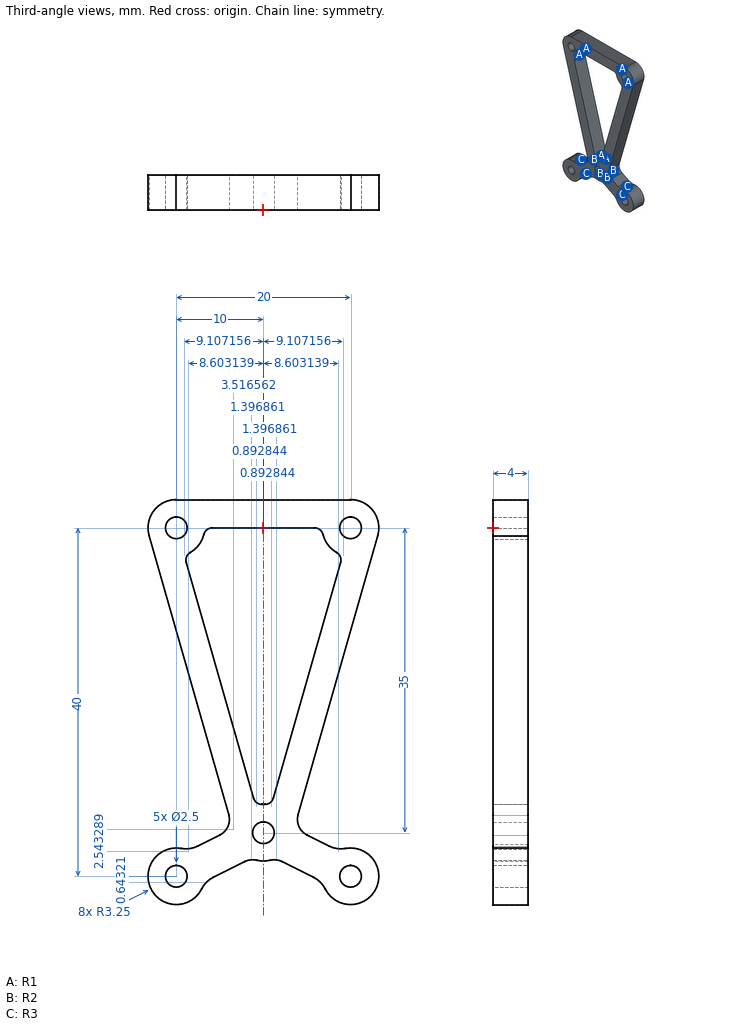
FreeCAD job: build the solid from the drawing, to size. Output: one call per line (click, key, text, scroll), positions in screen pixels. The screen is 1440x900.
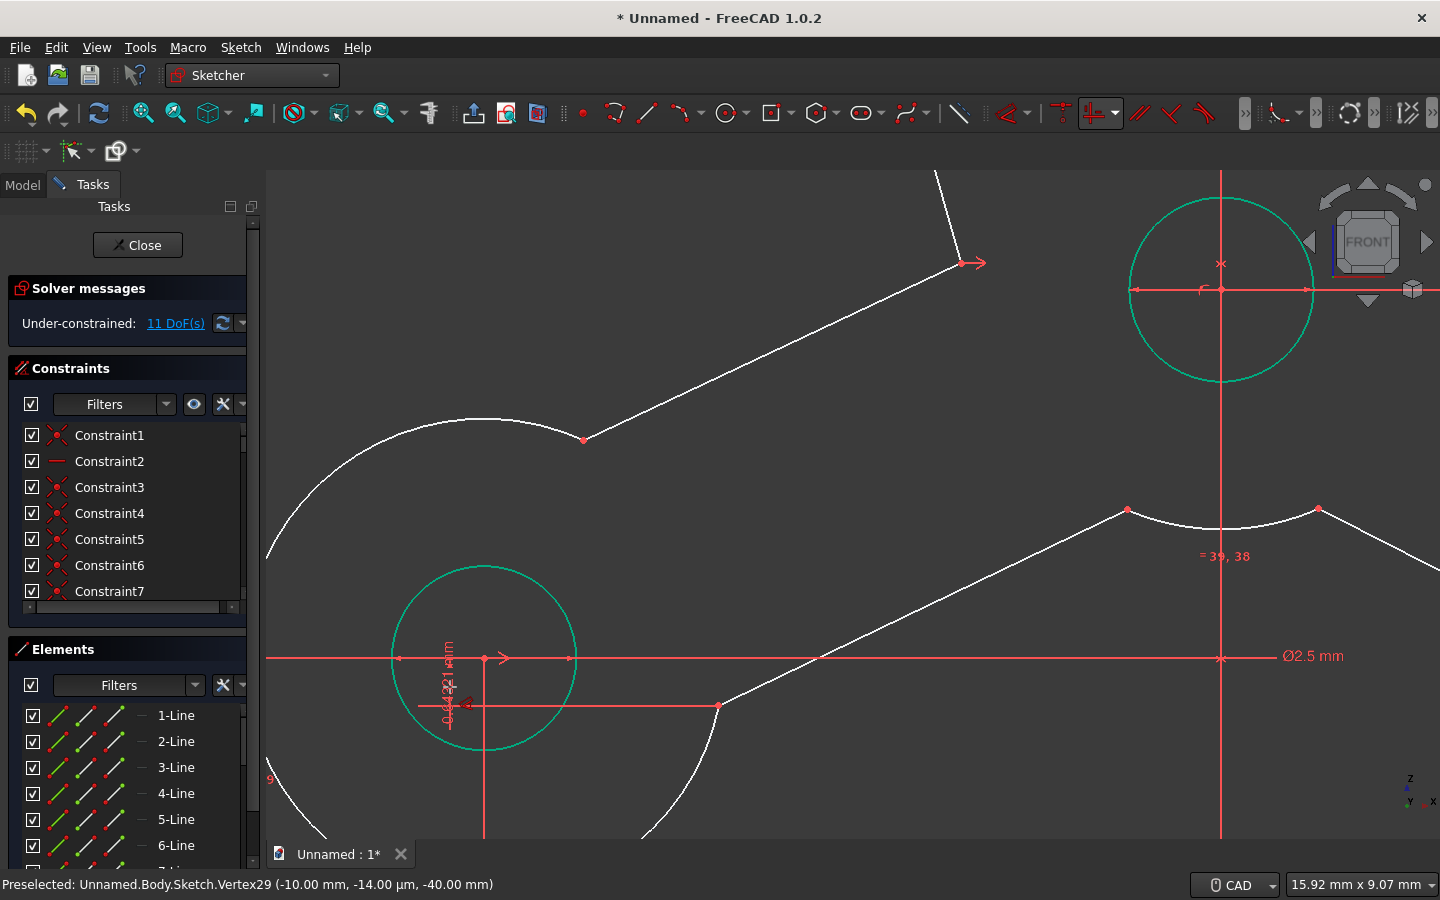
scroll(716, 722, down, 10)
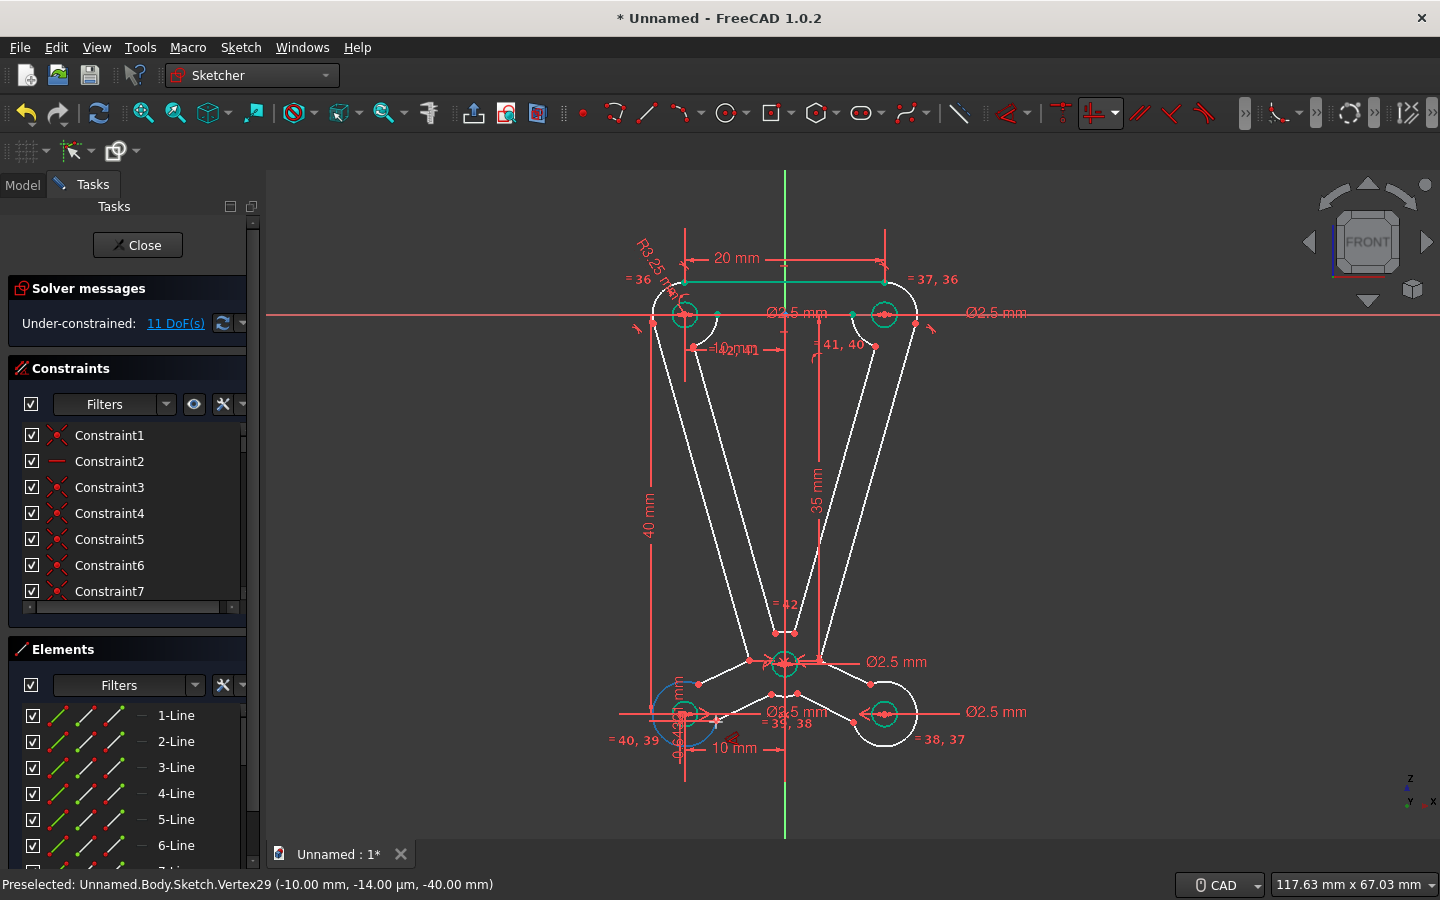
scroll(853, 722, up, 10)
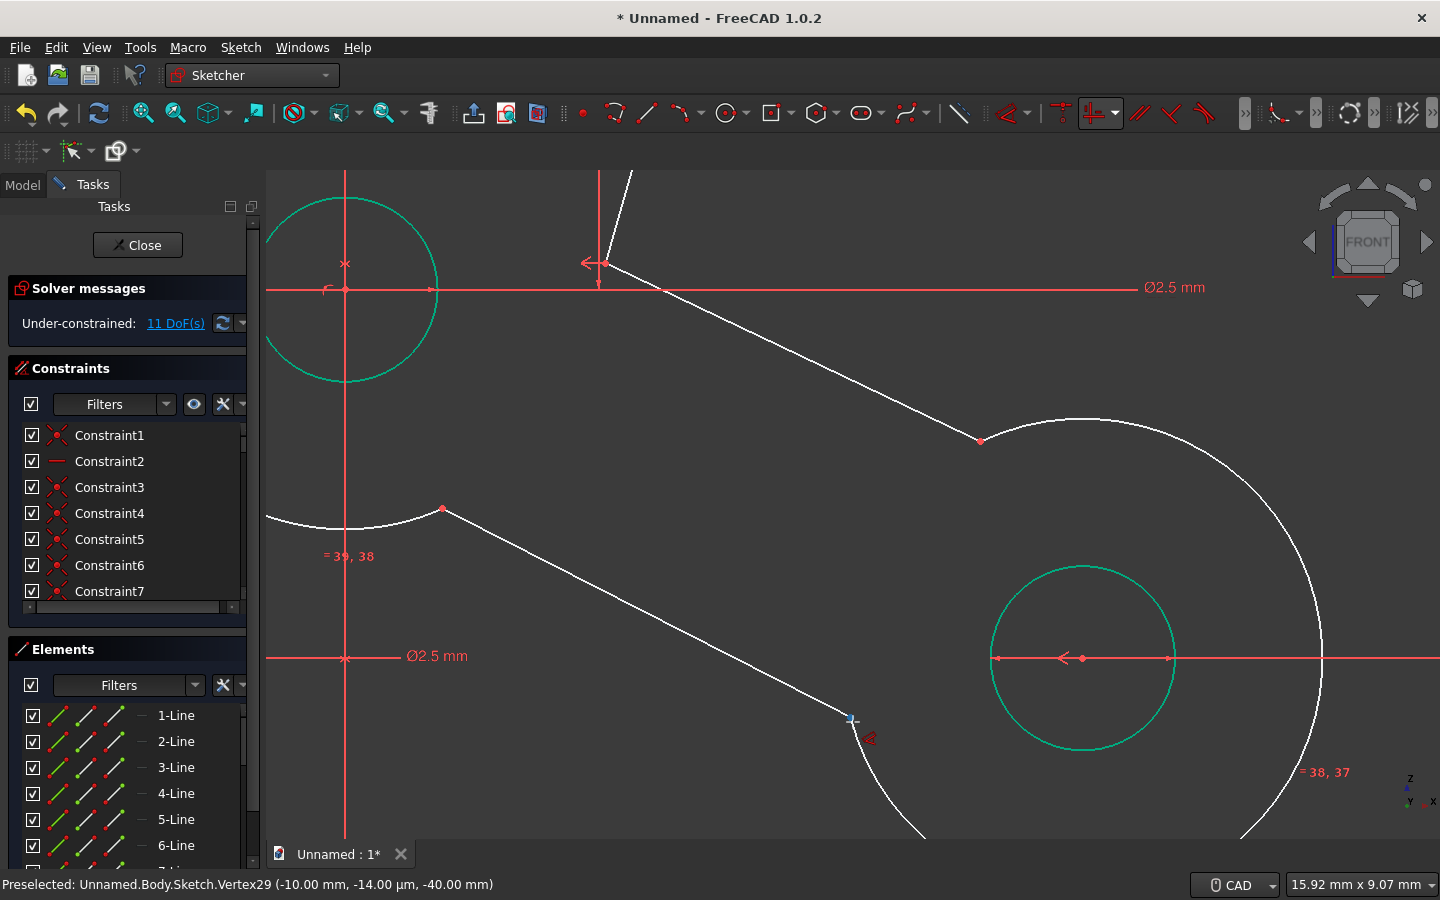
click(851, 717)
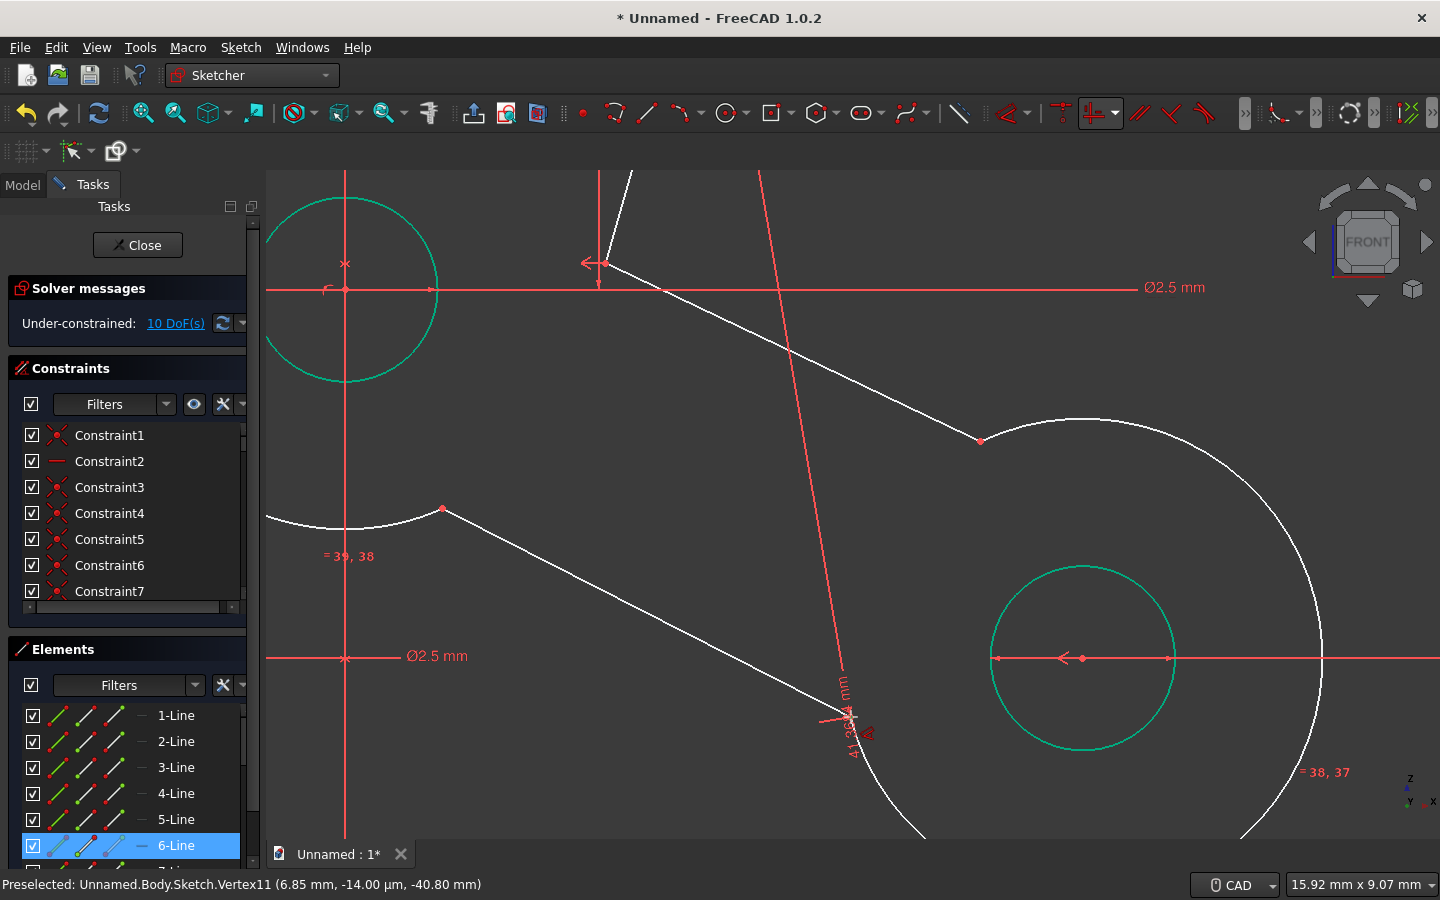
click(1083, 658)
click(1117, 688)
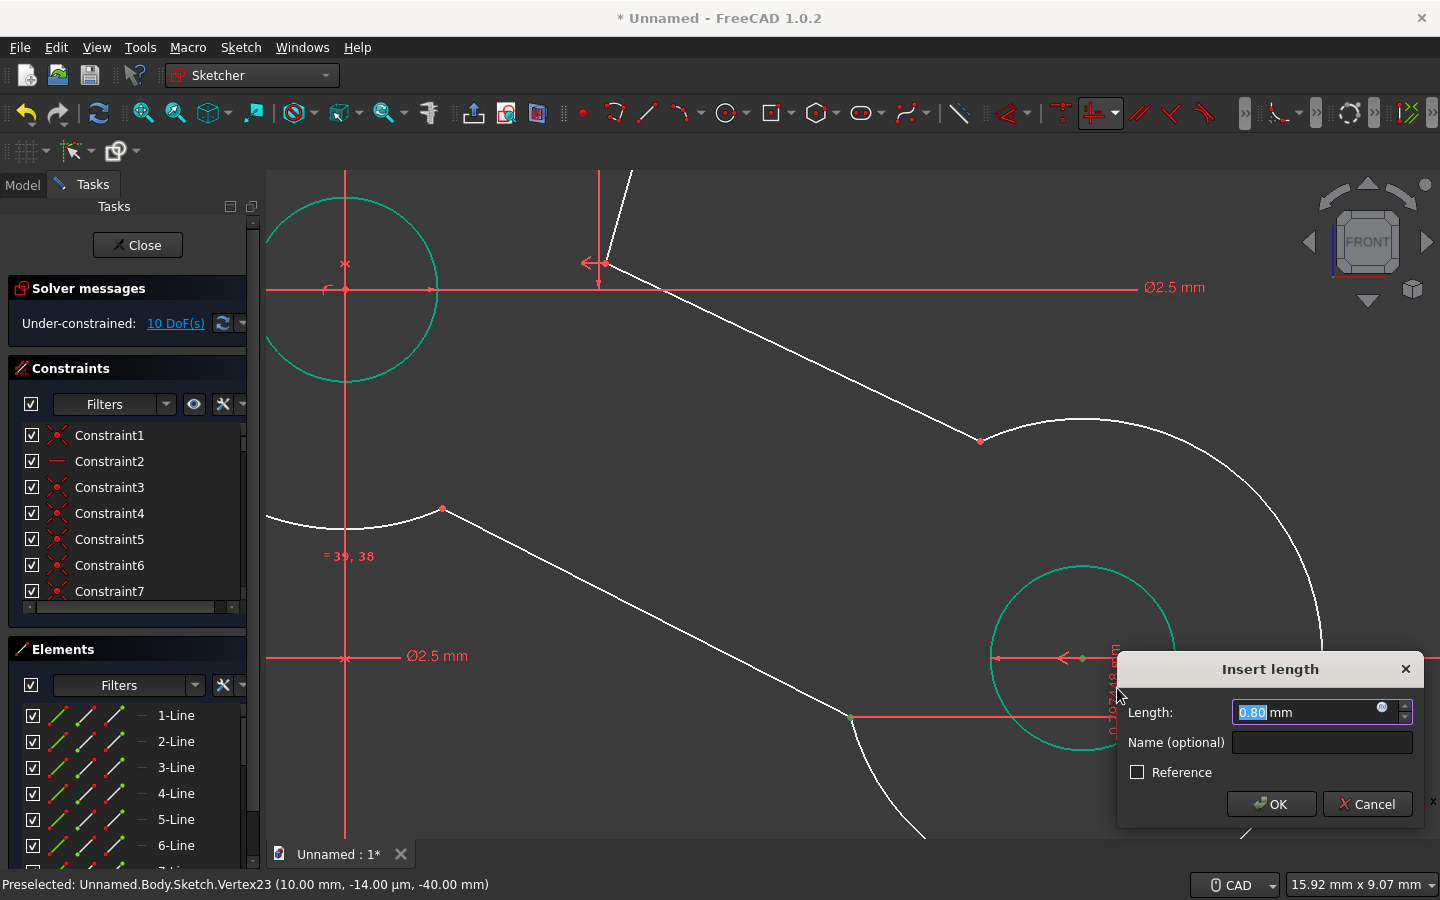
text(0.64321)
key(Return)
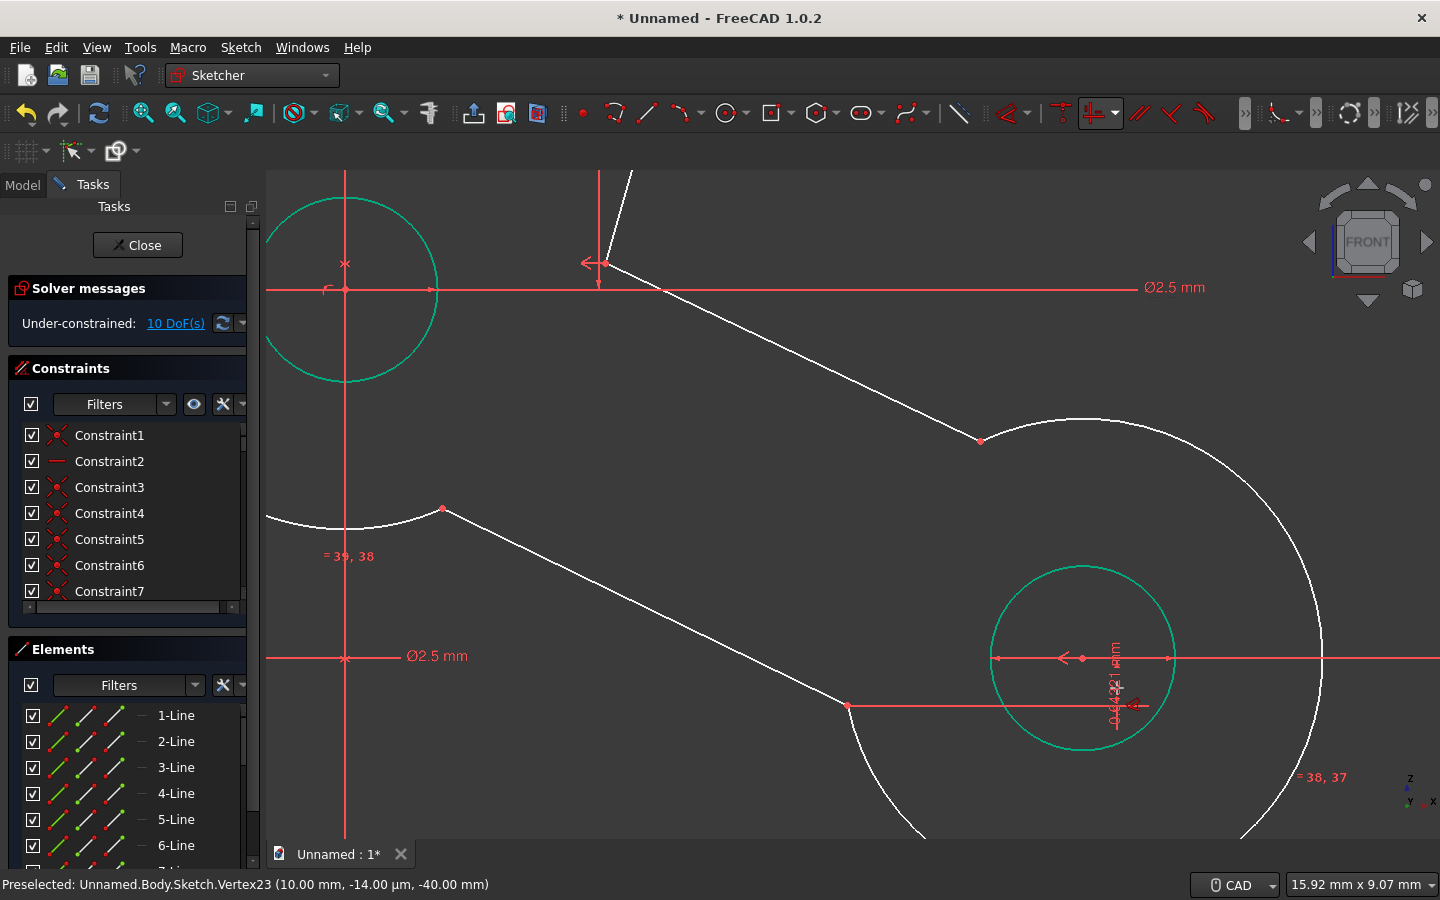
scroll(853, 722, down, 10)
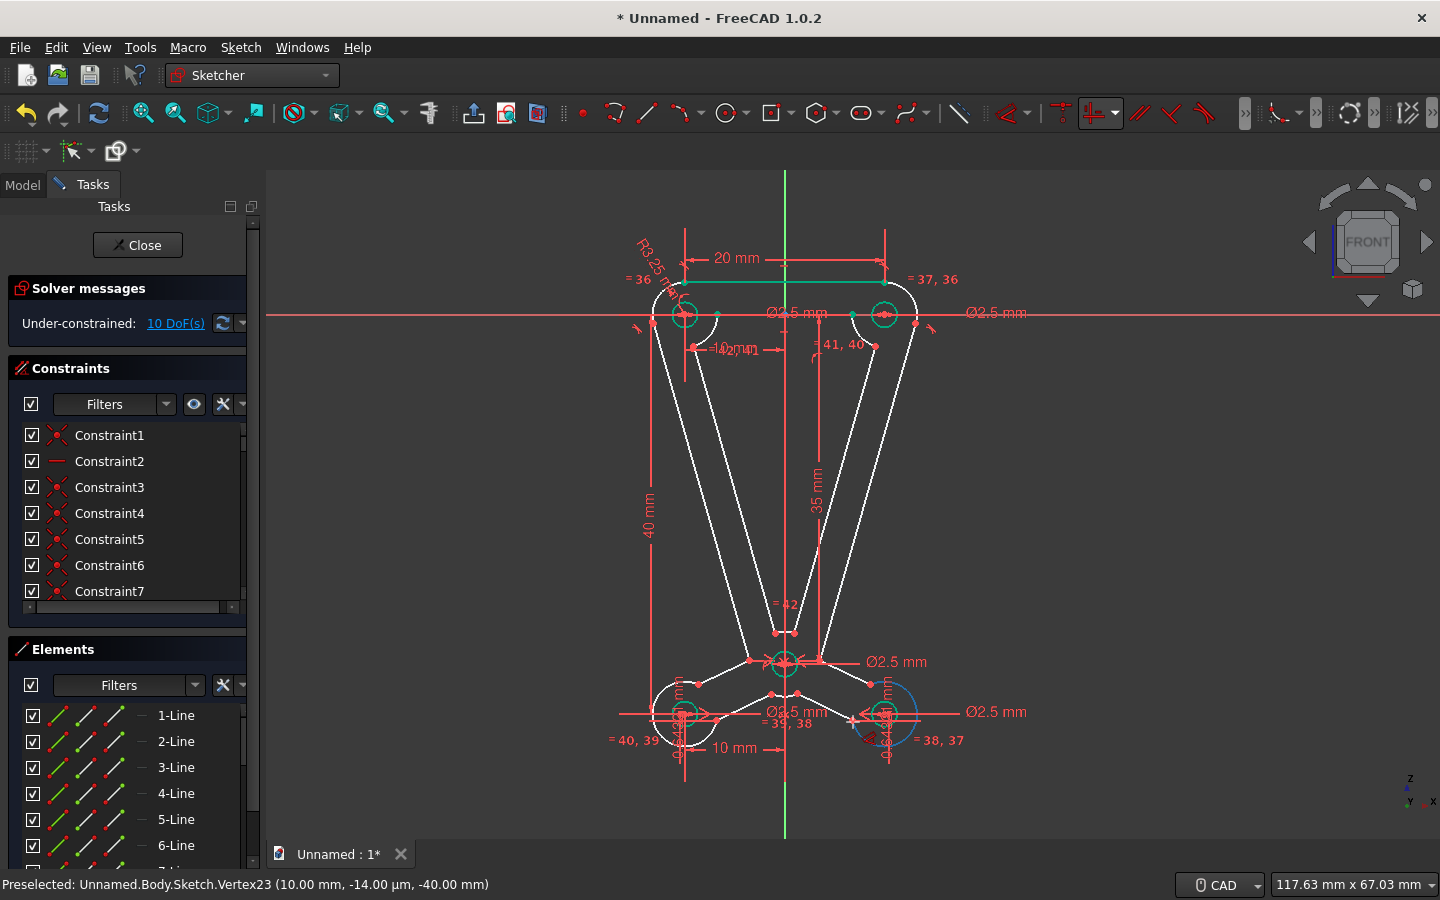
click(698, 685)
click(761, 719)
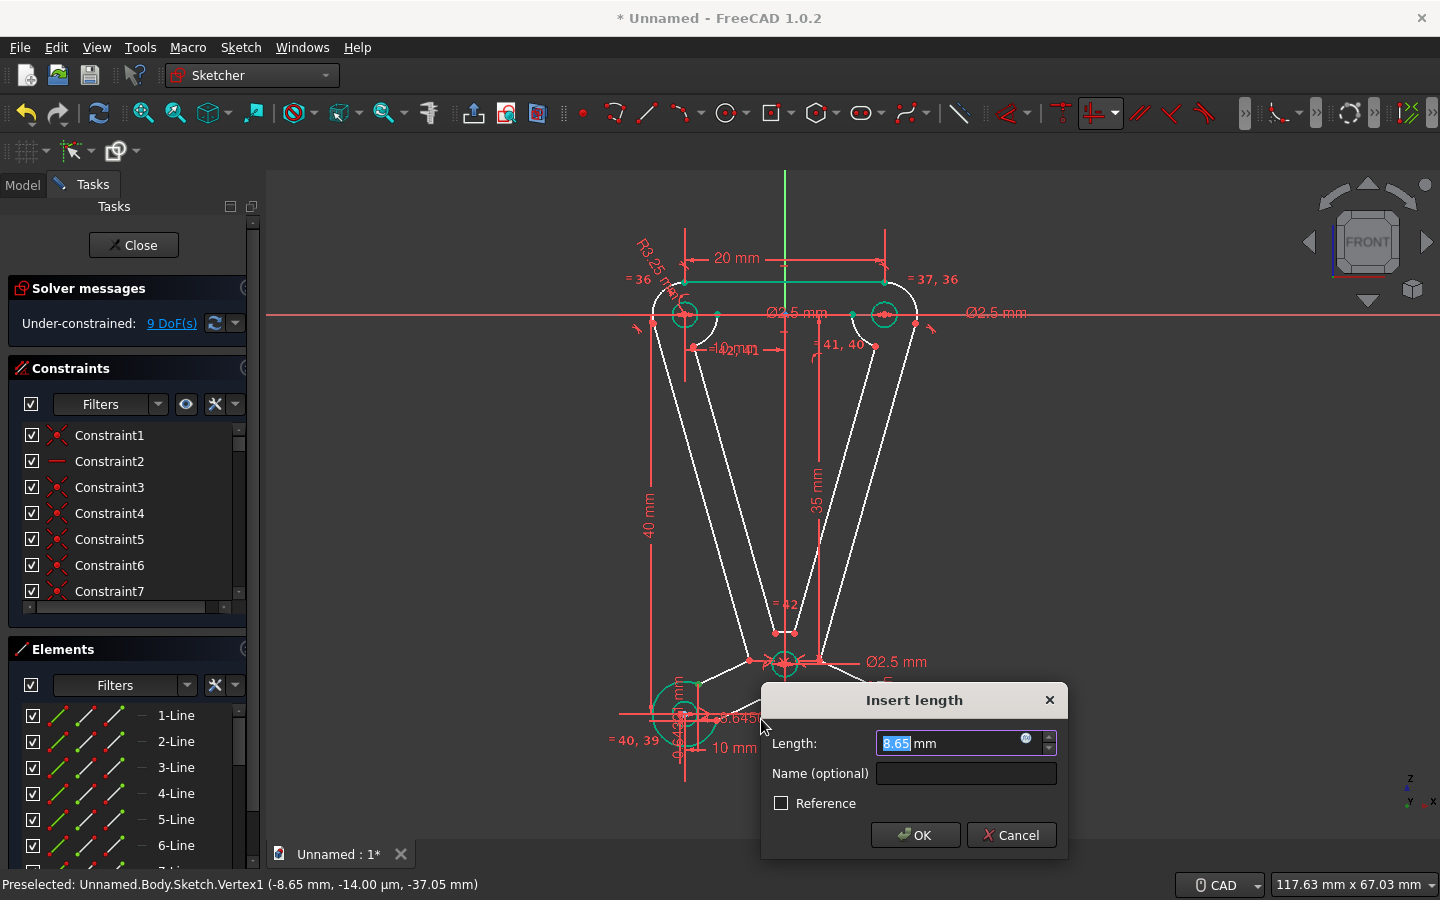
text(8.603139)
key(Return)